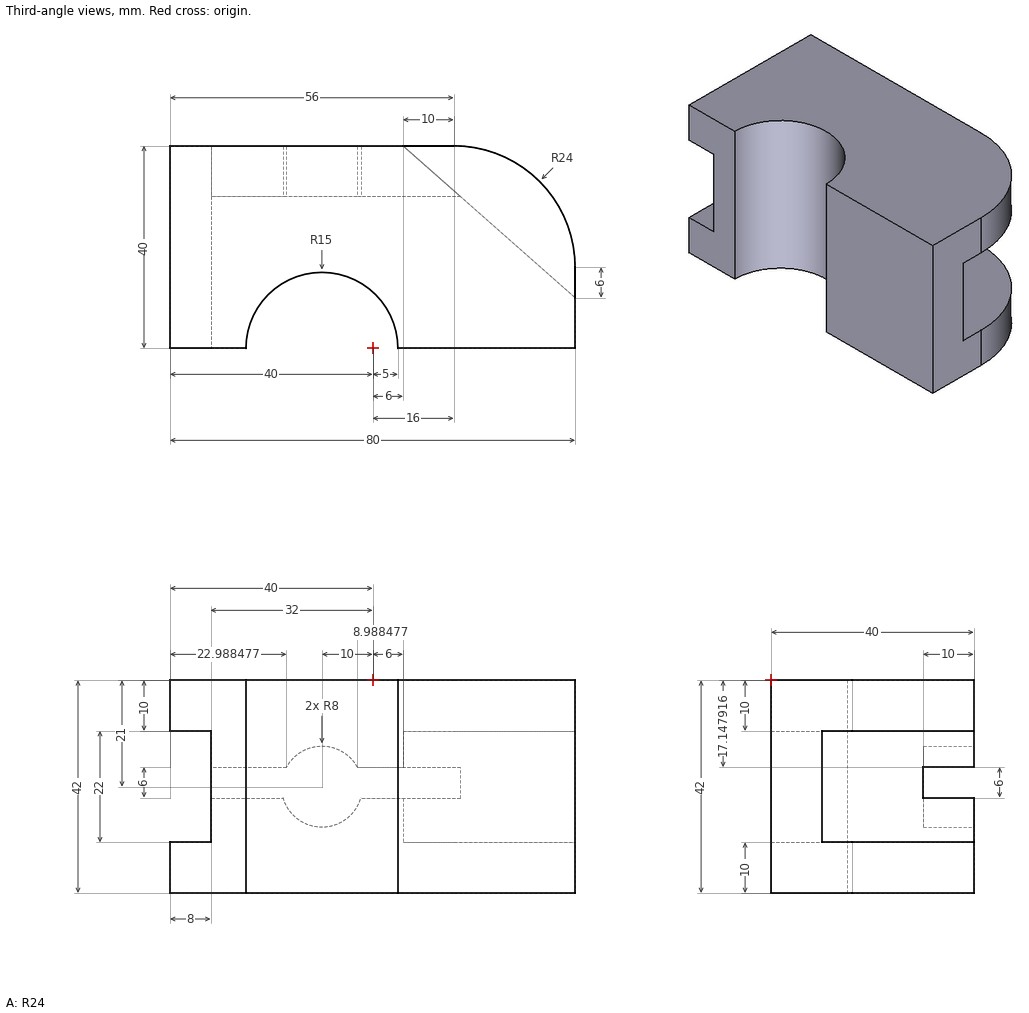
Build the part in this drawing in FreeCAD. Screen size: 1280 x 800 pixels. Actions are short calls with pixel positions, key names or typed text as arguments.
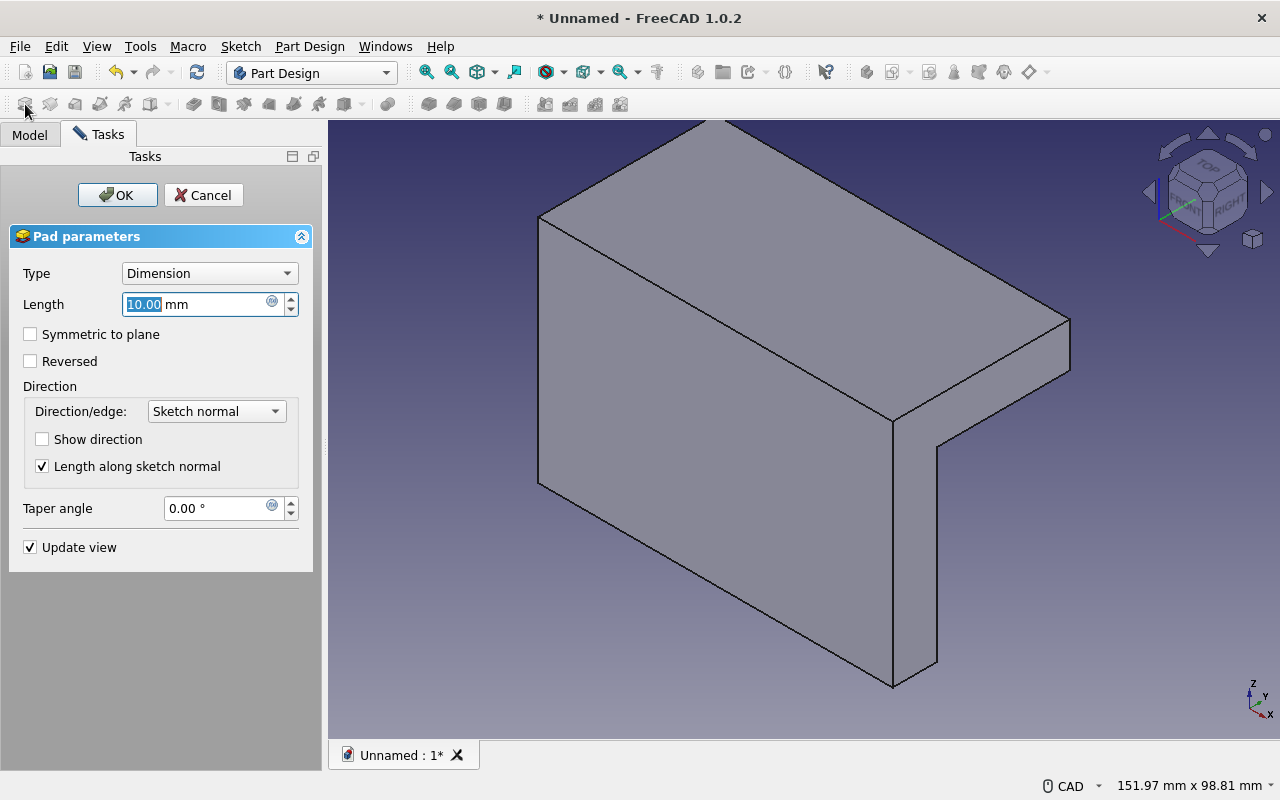
text(10)
key(Tab)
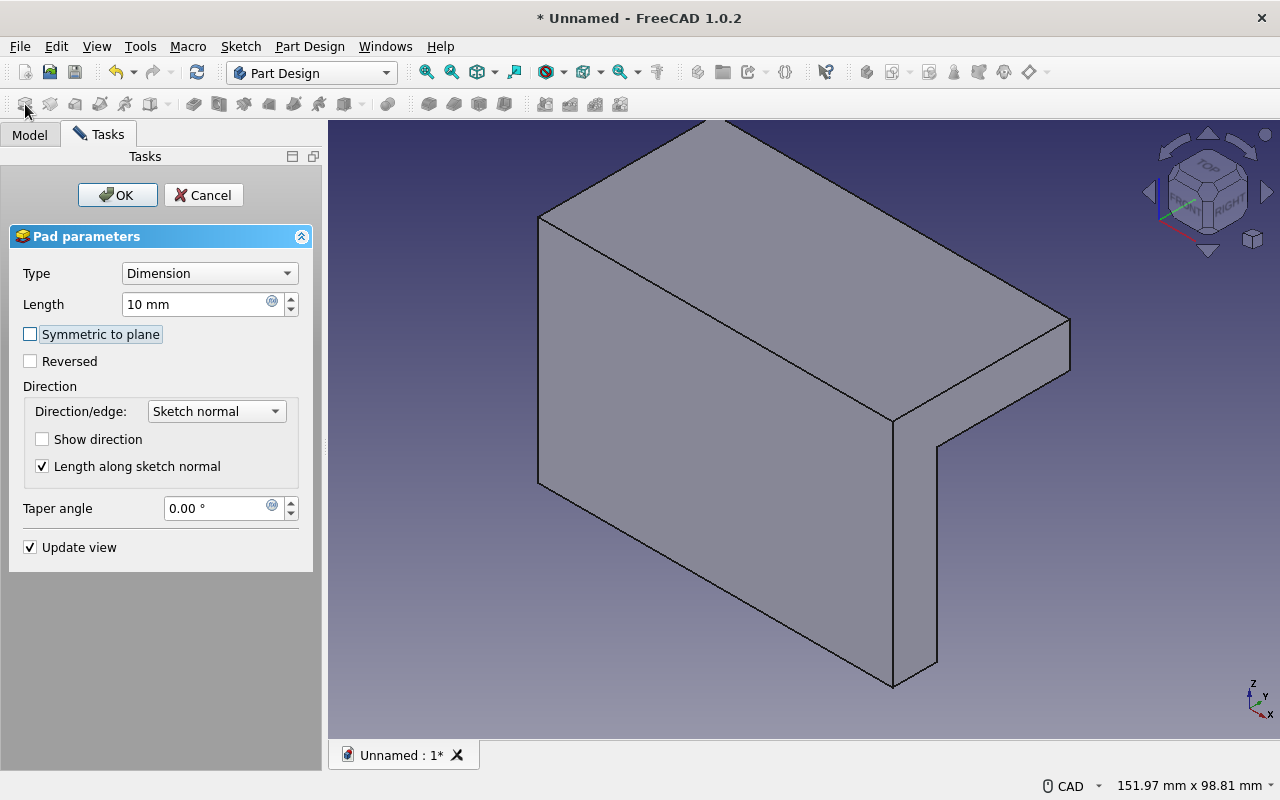
click(31, 361)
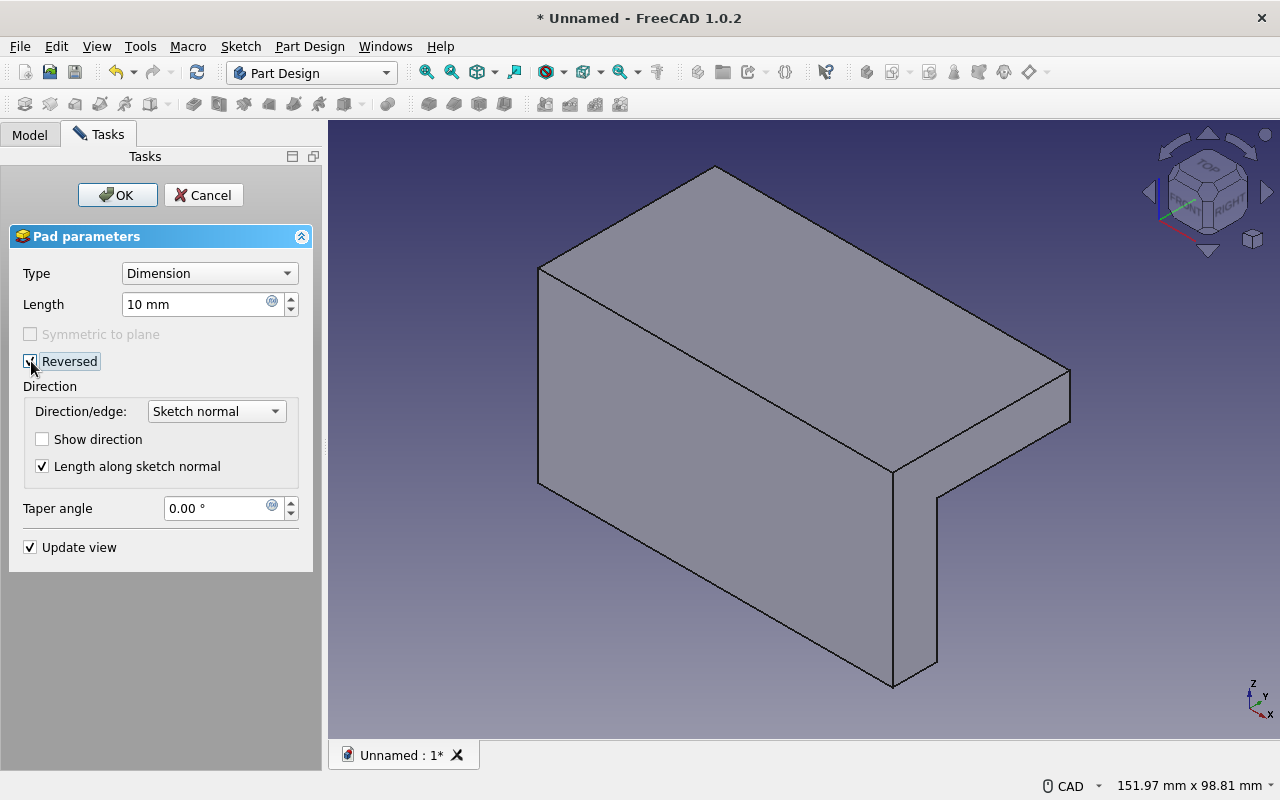
click(118, 195)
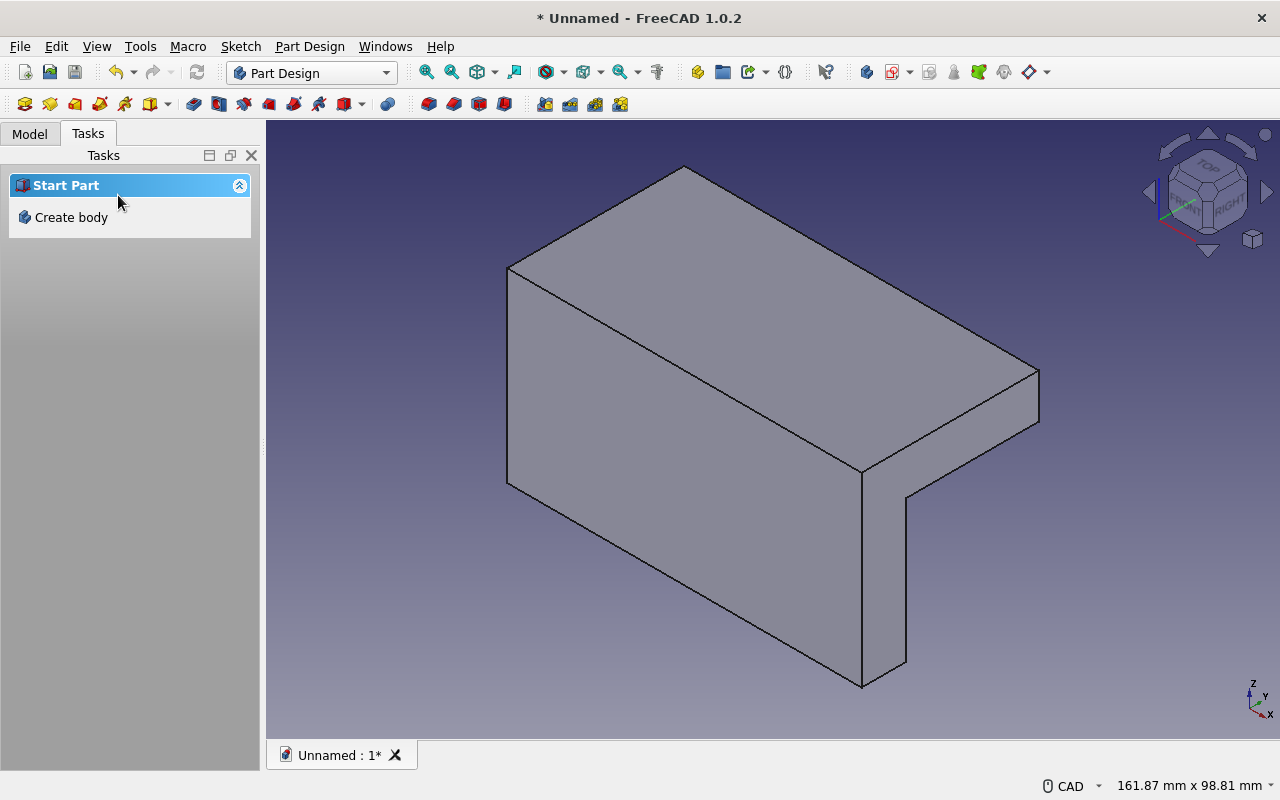
key(5)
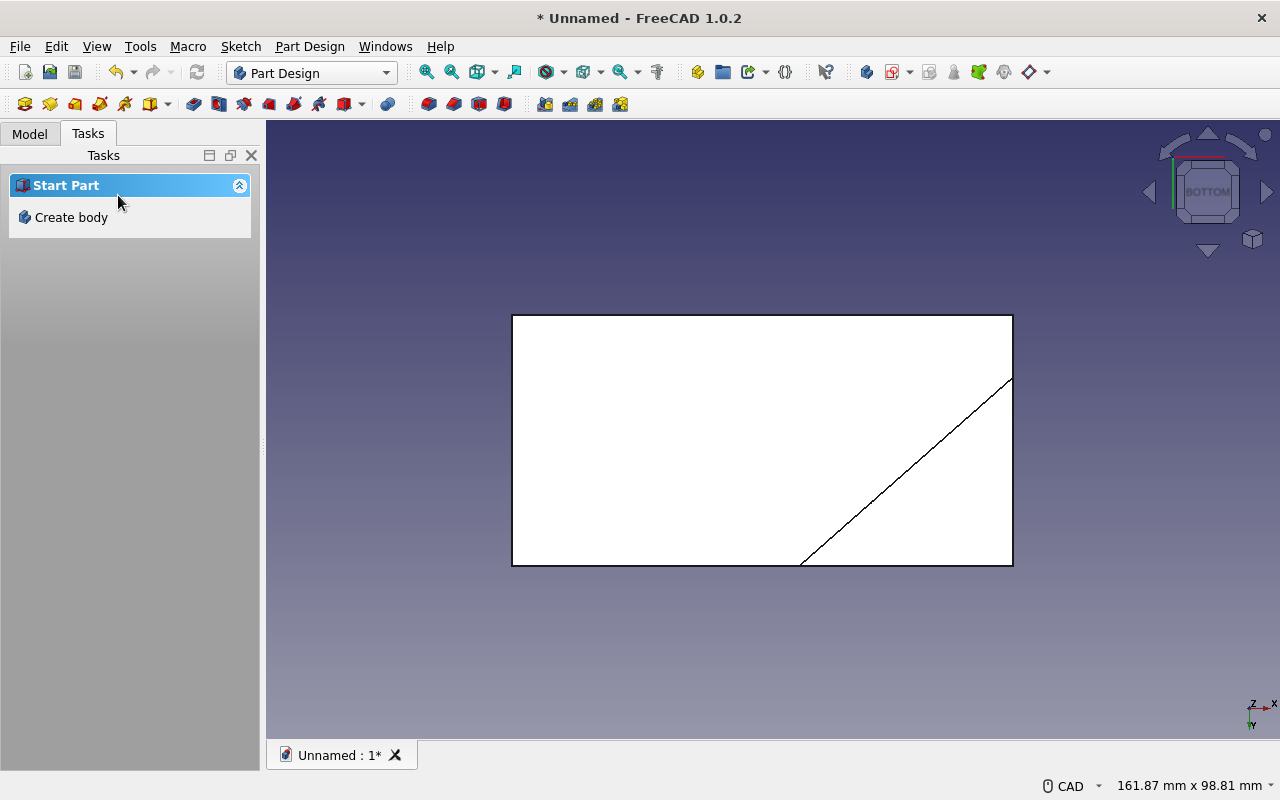
click(691, 439)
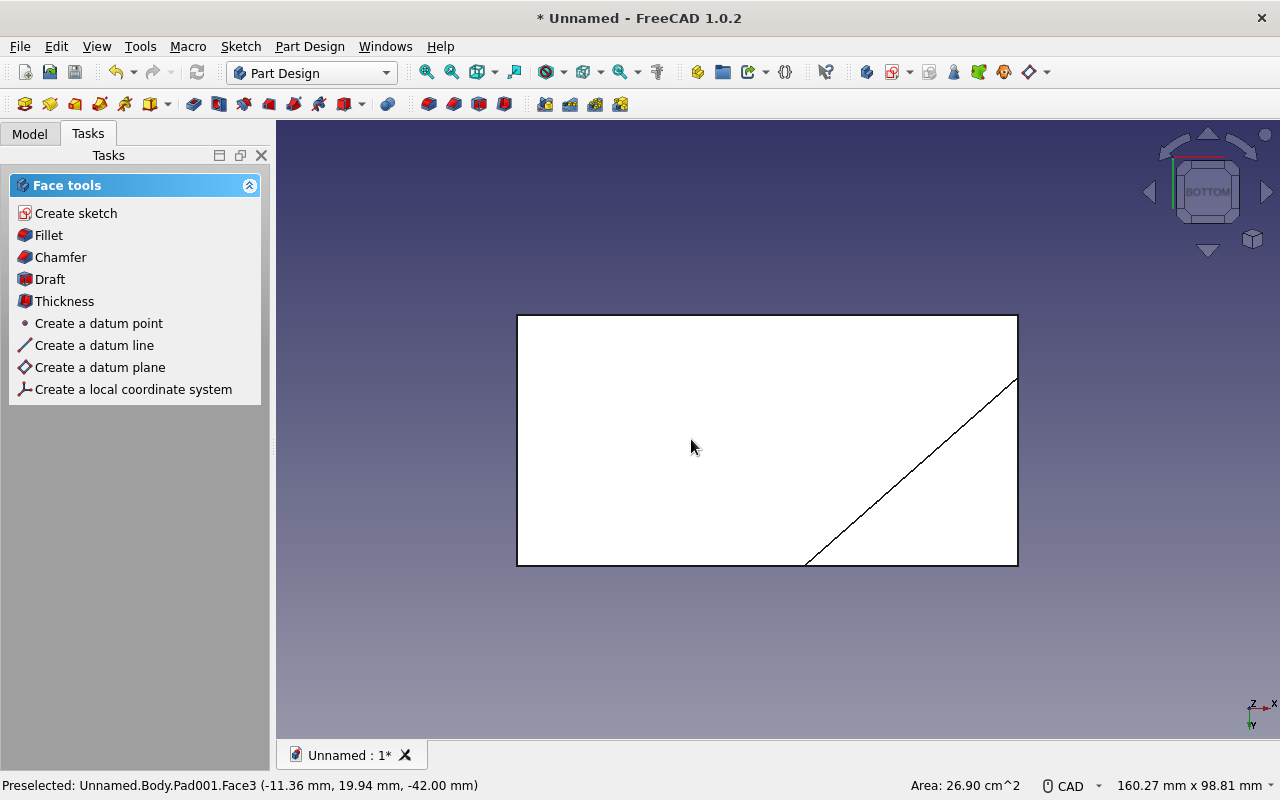
click(892, 72)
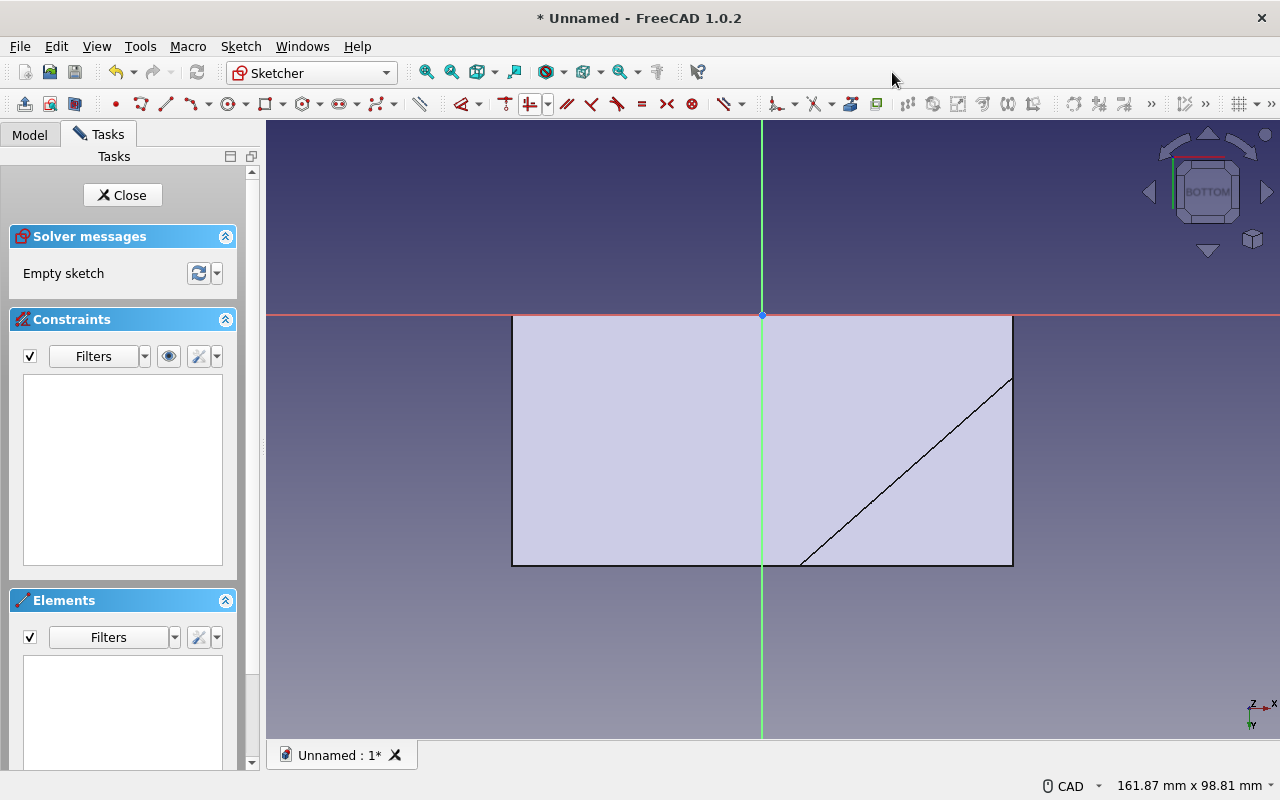
click(264, 104)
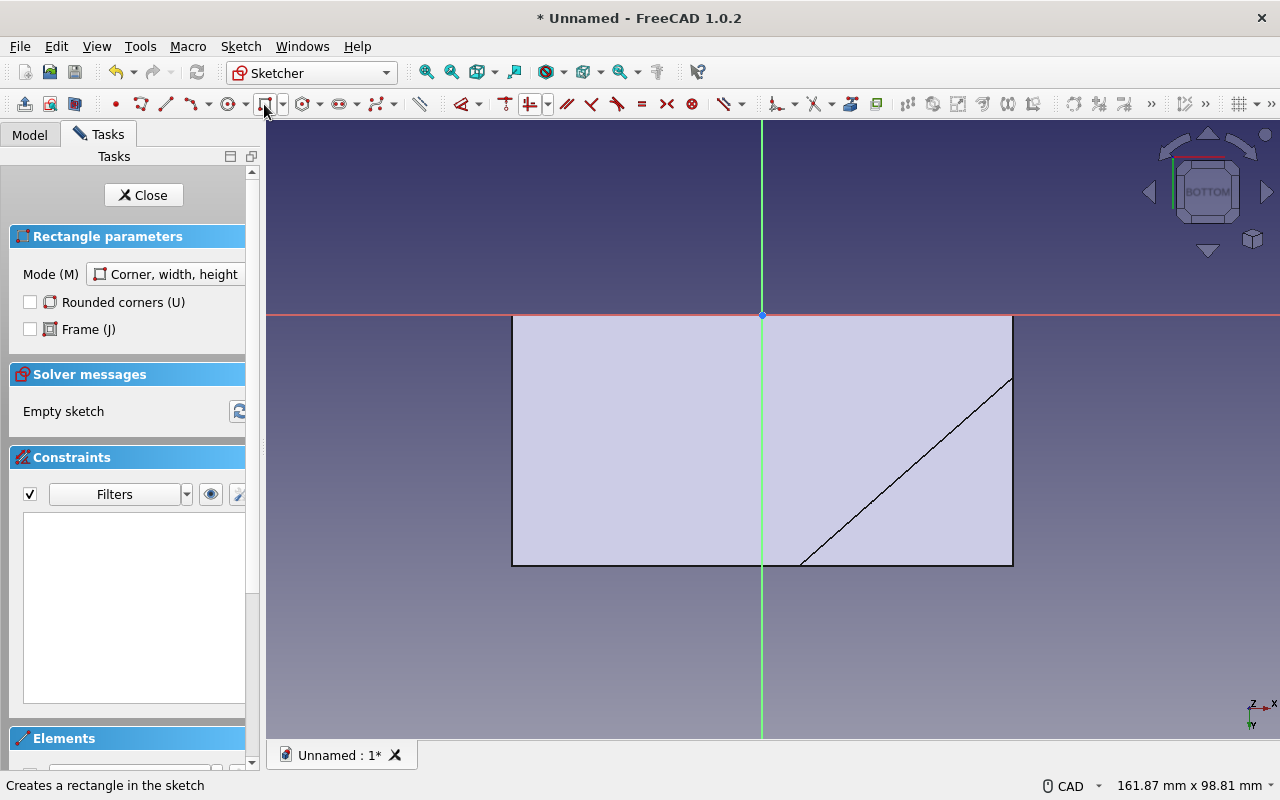
click(512, 315)
move(1013, 566)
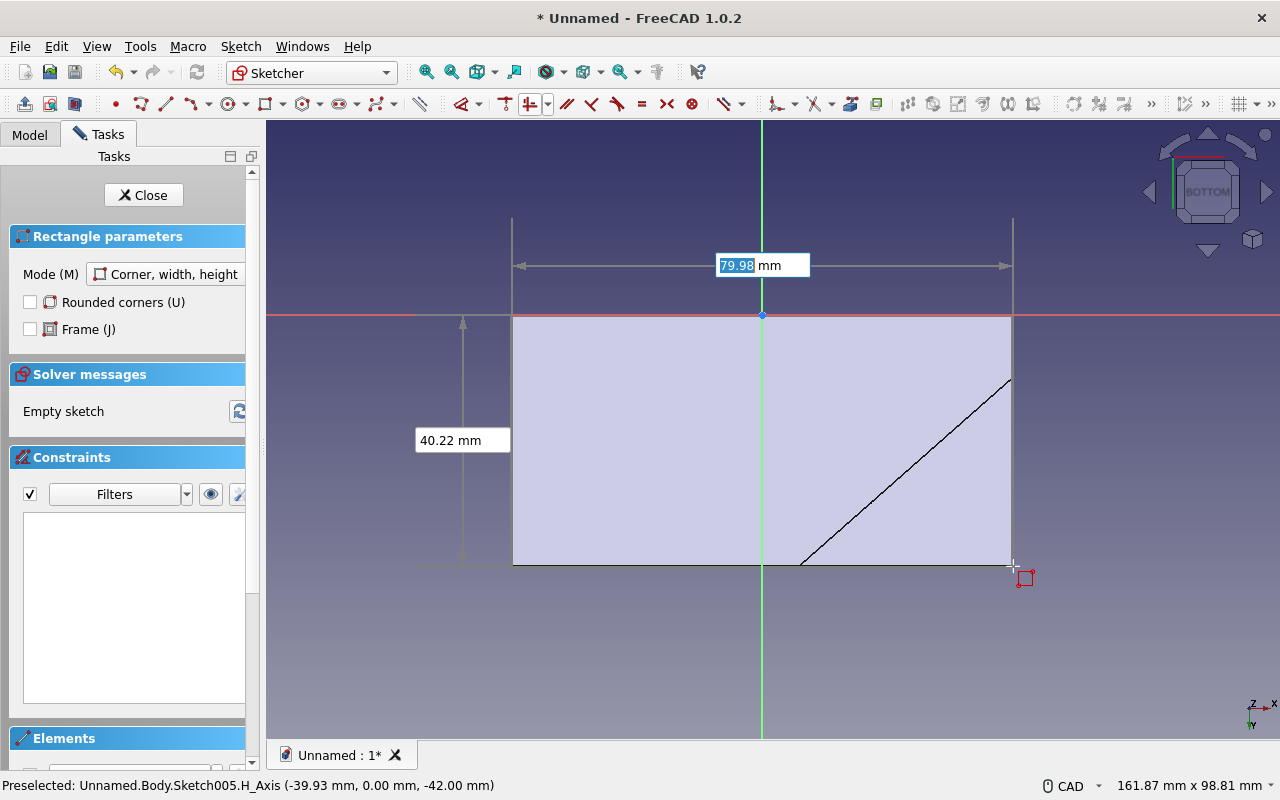
text(80)
key(Tab)
text(40)
key(Return)
key(Escape)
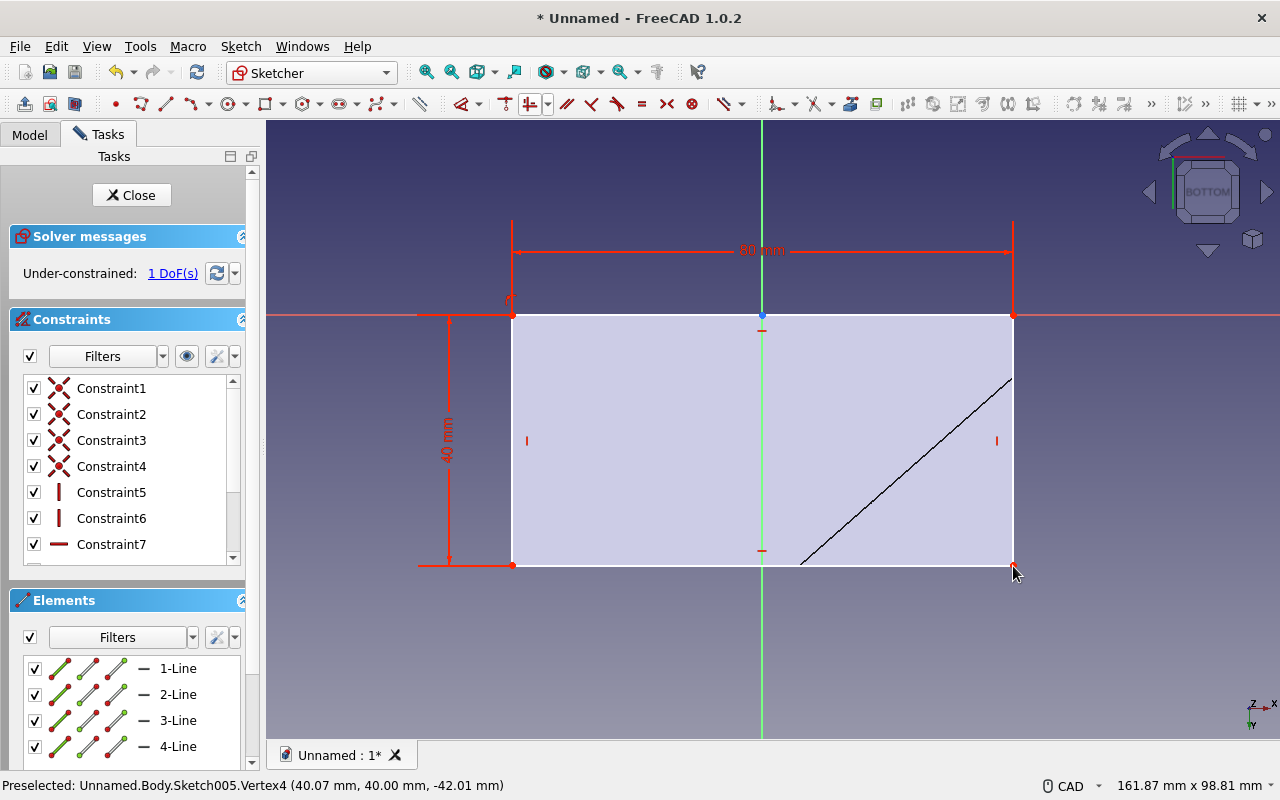
key(d)